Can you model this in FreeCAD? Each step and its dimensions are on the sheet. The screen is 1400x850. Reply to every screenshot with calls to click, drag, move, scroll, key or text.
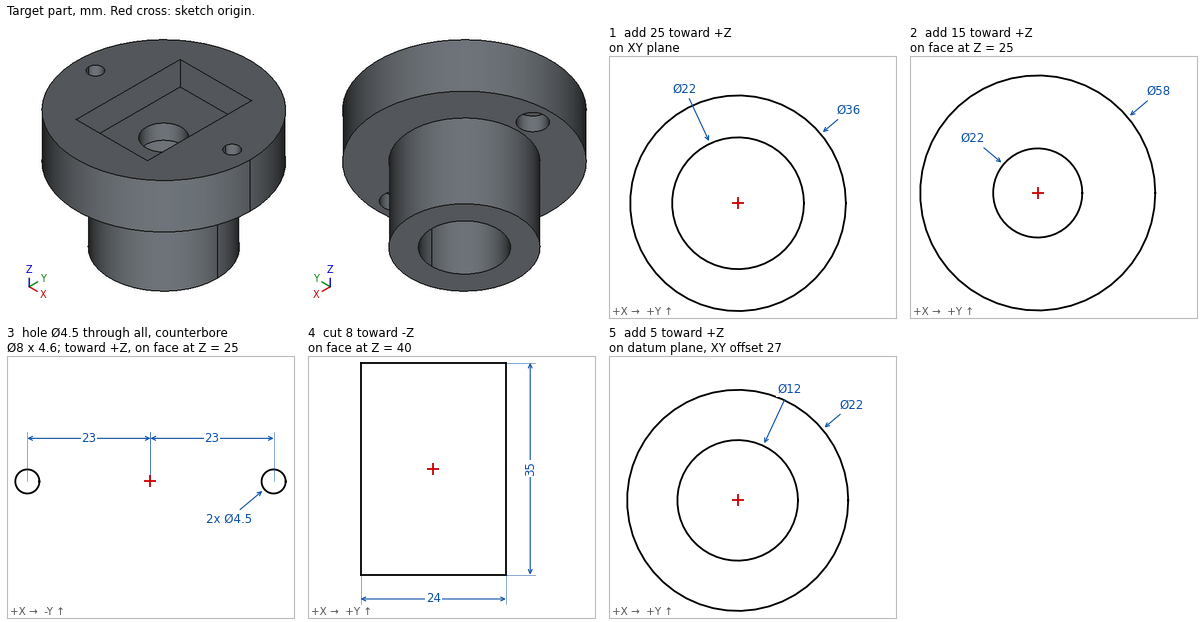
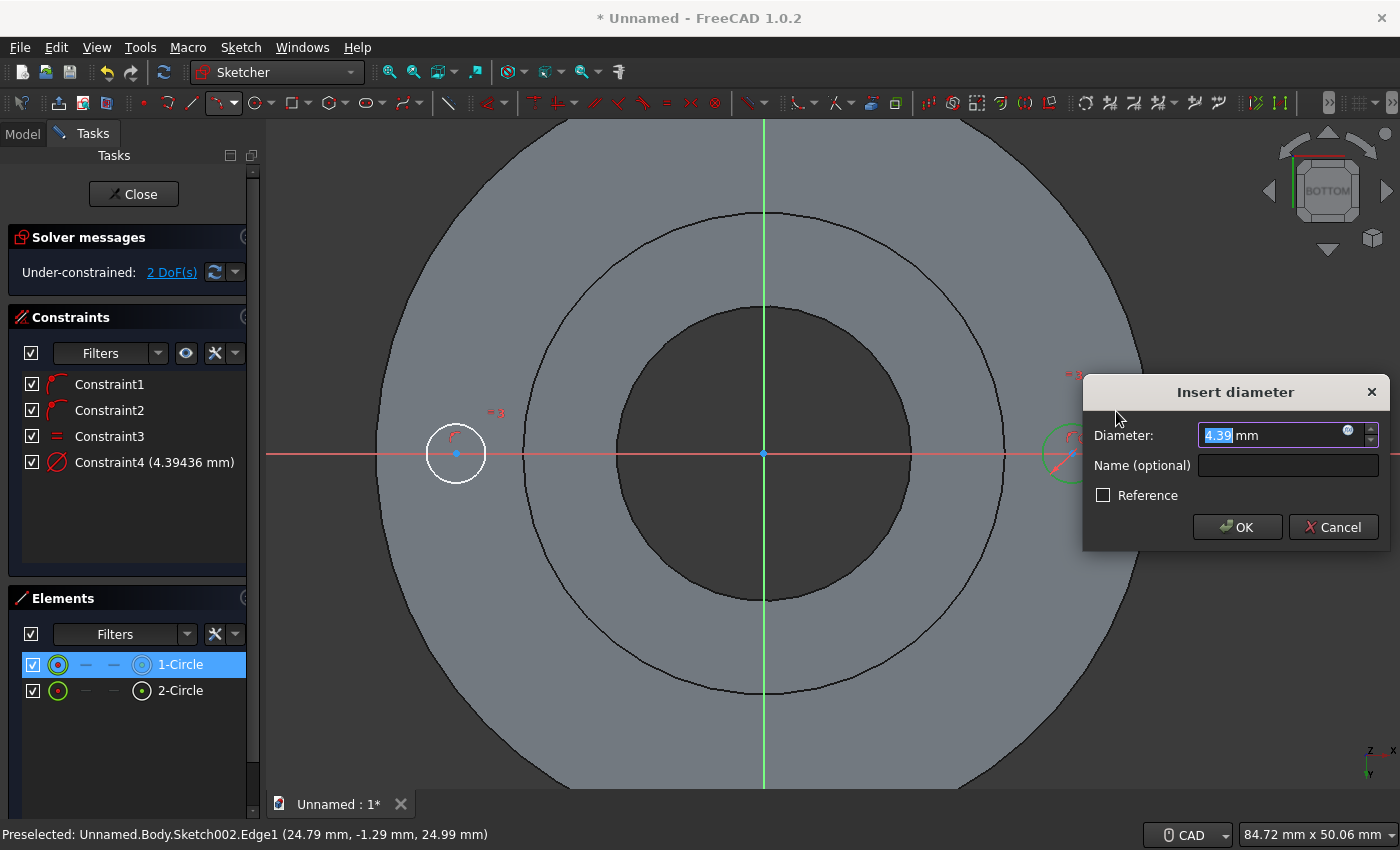
text(4.5)
key(Return)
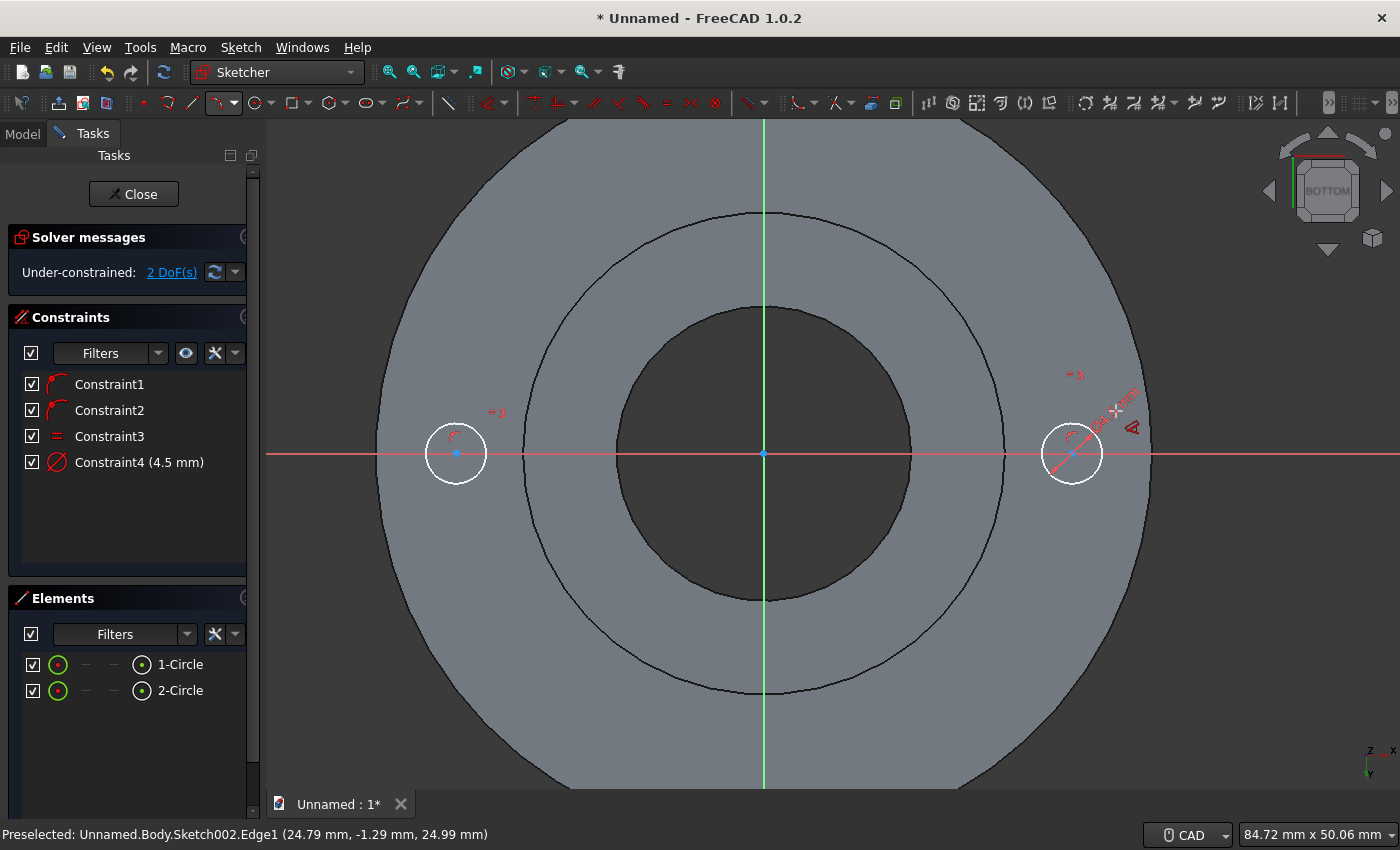
click(1072, 454)
click(918, 488)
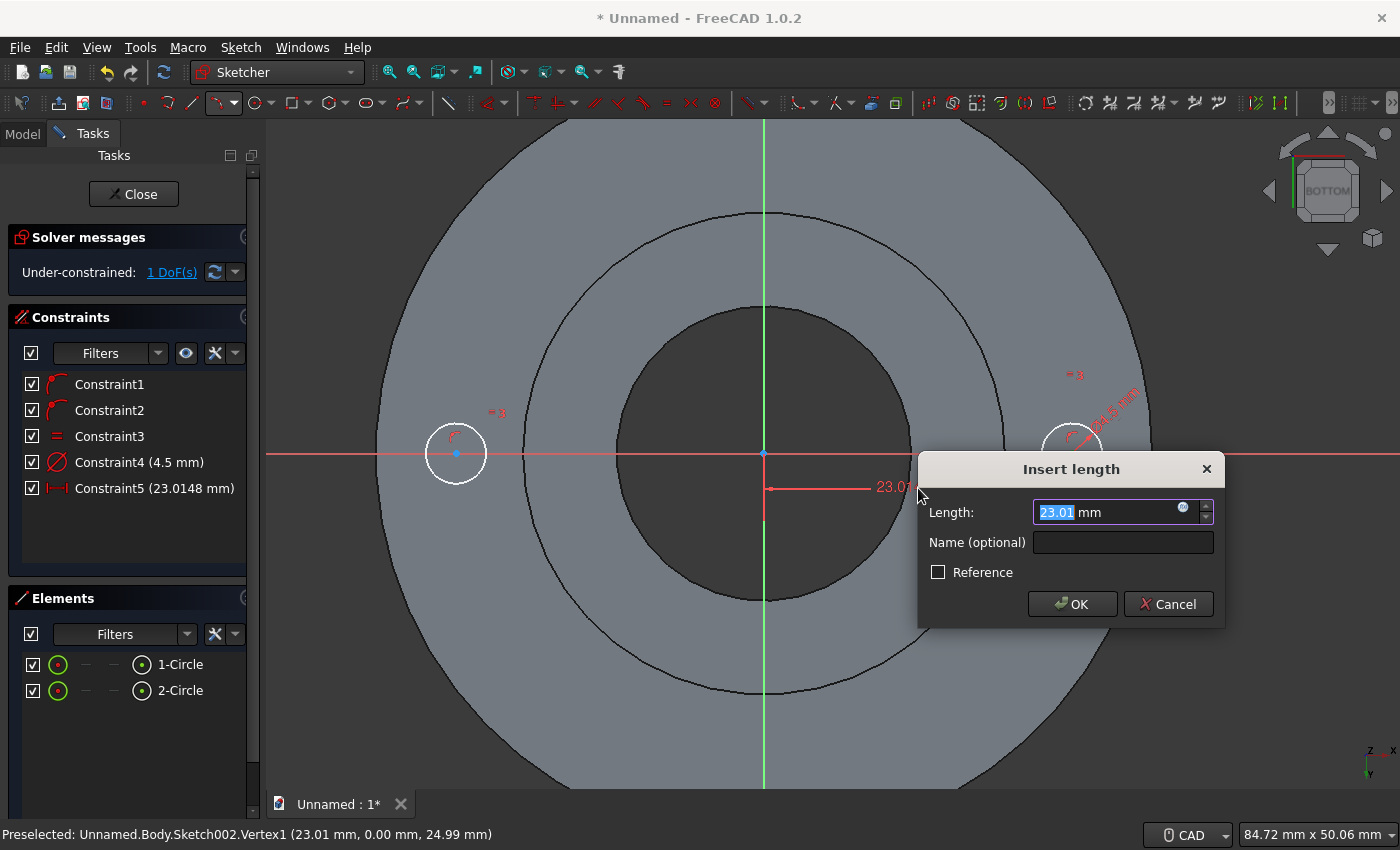
text(23)
key(Return)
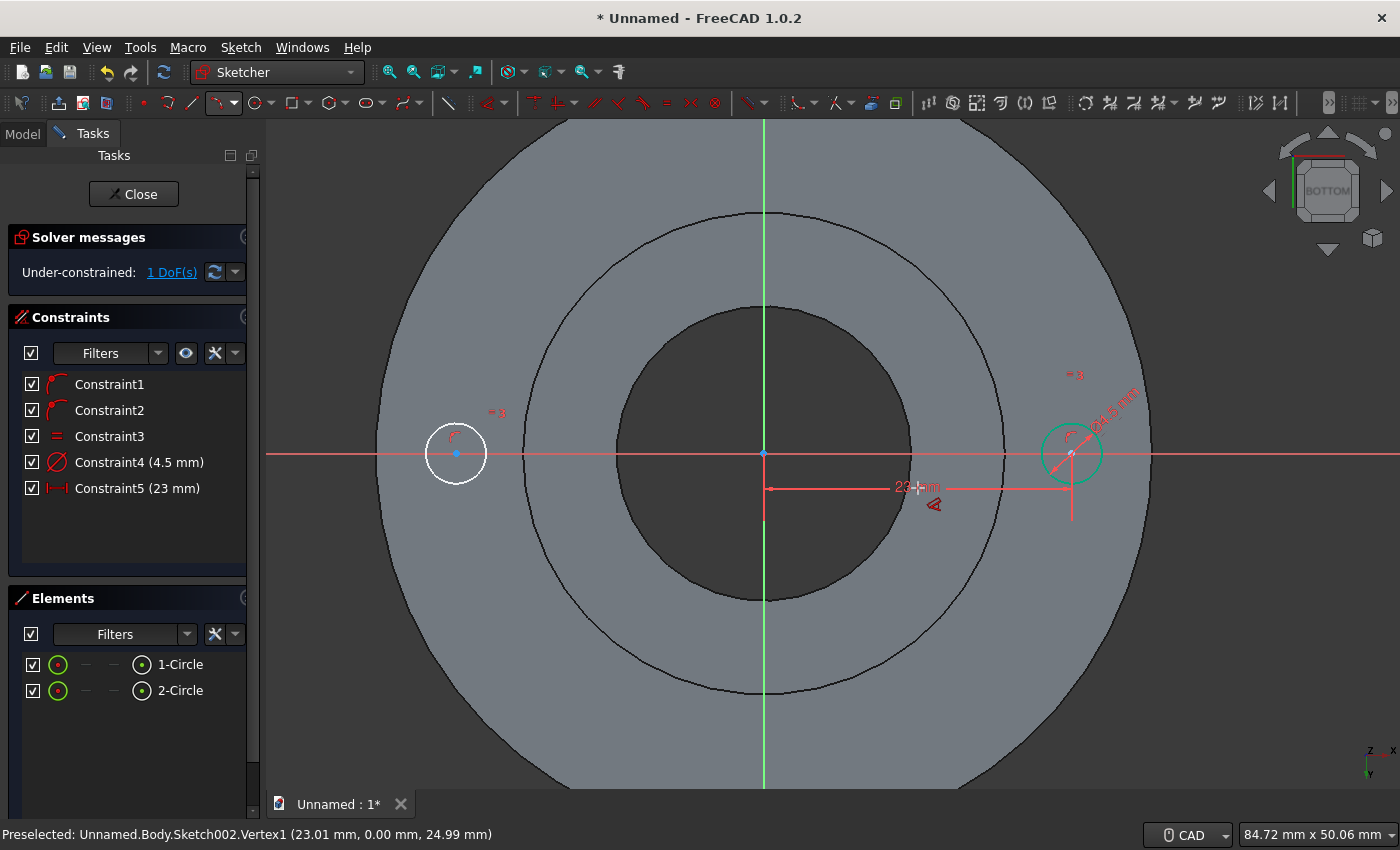
click(456, 454)
click(610, 488)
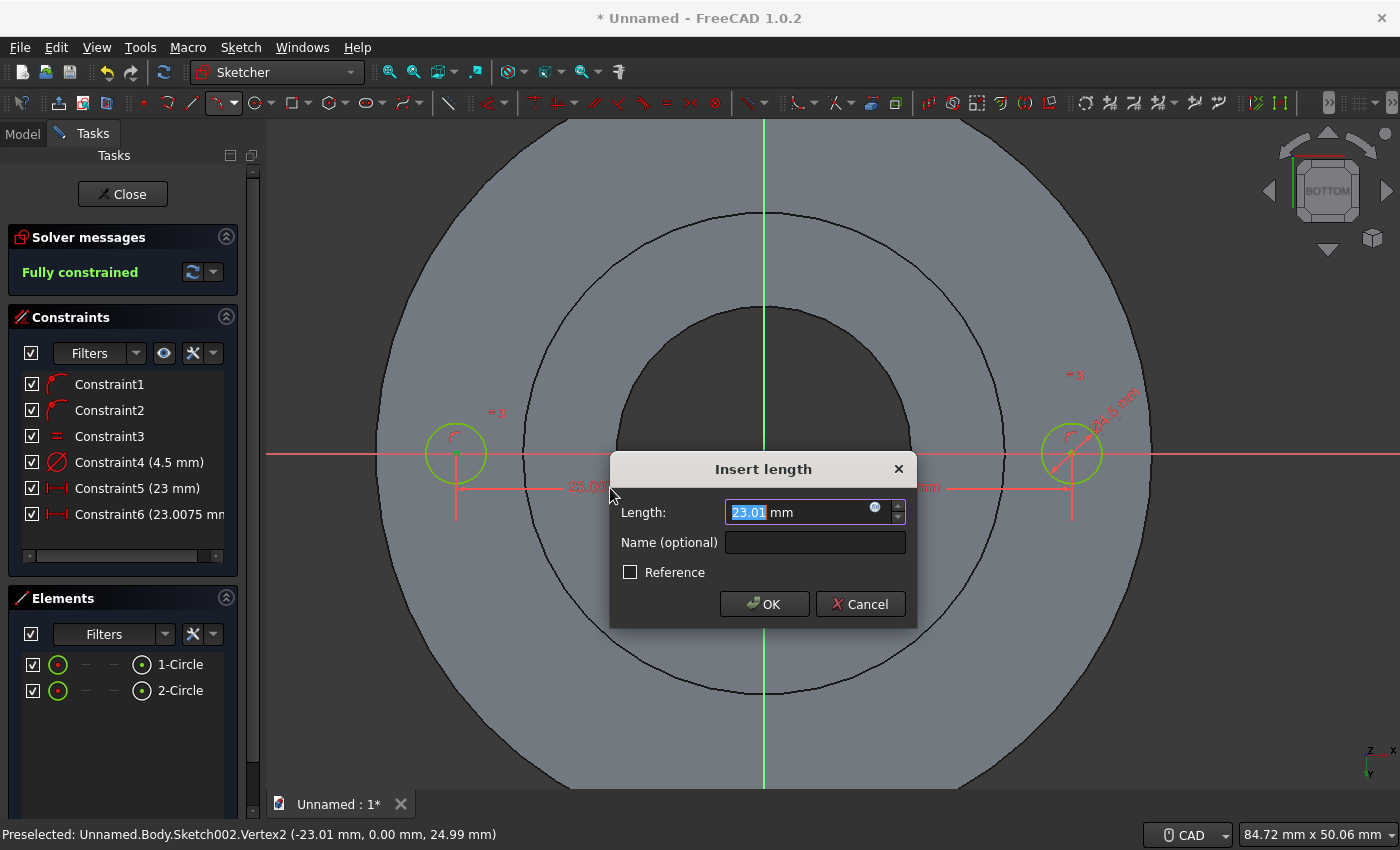
text(23)
key(Return)
key(Escape)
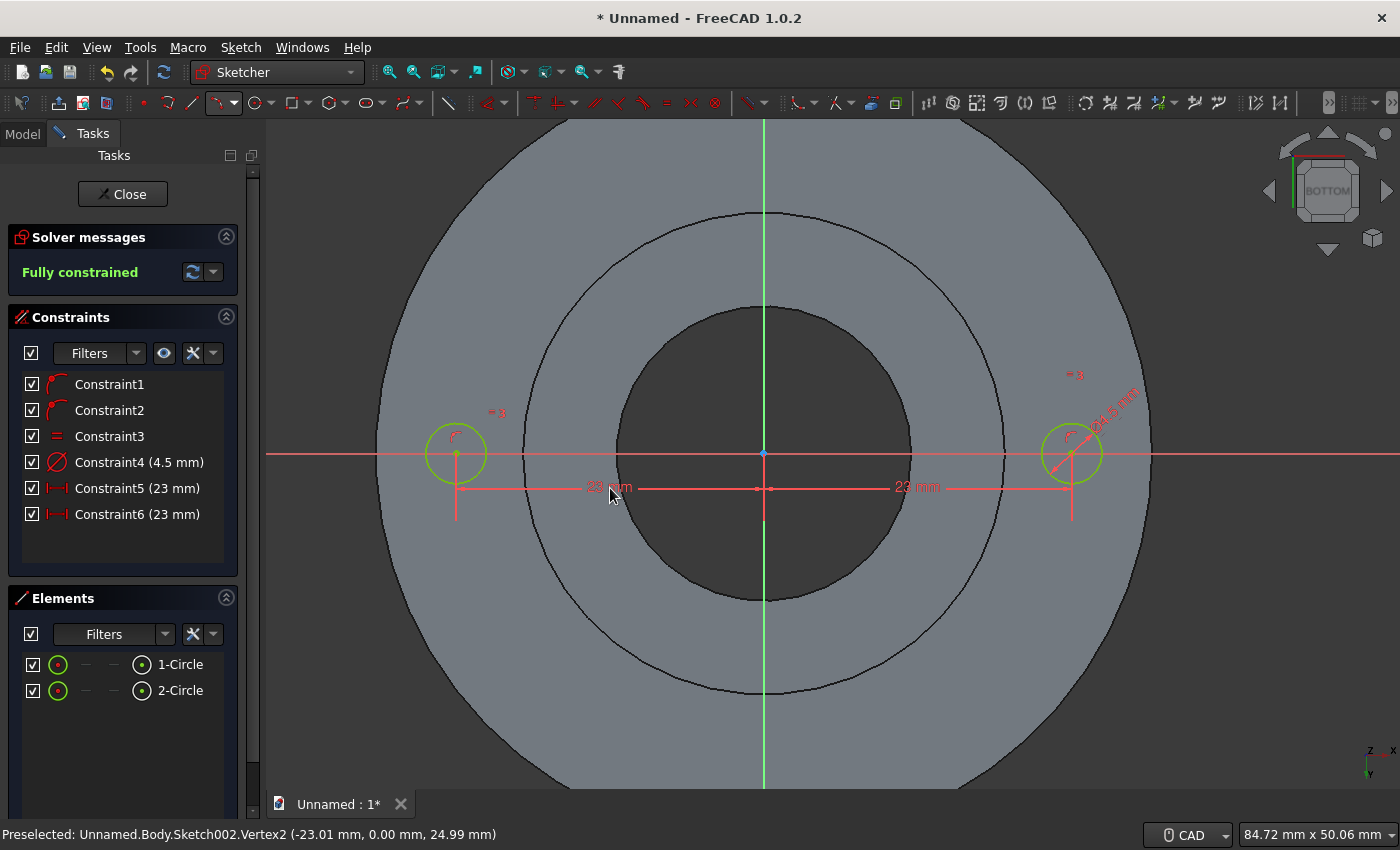
click(123, 194)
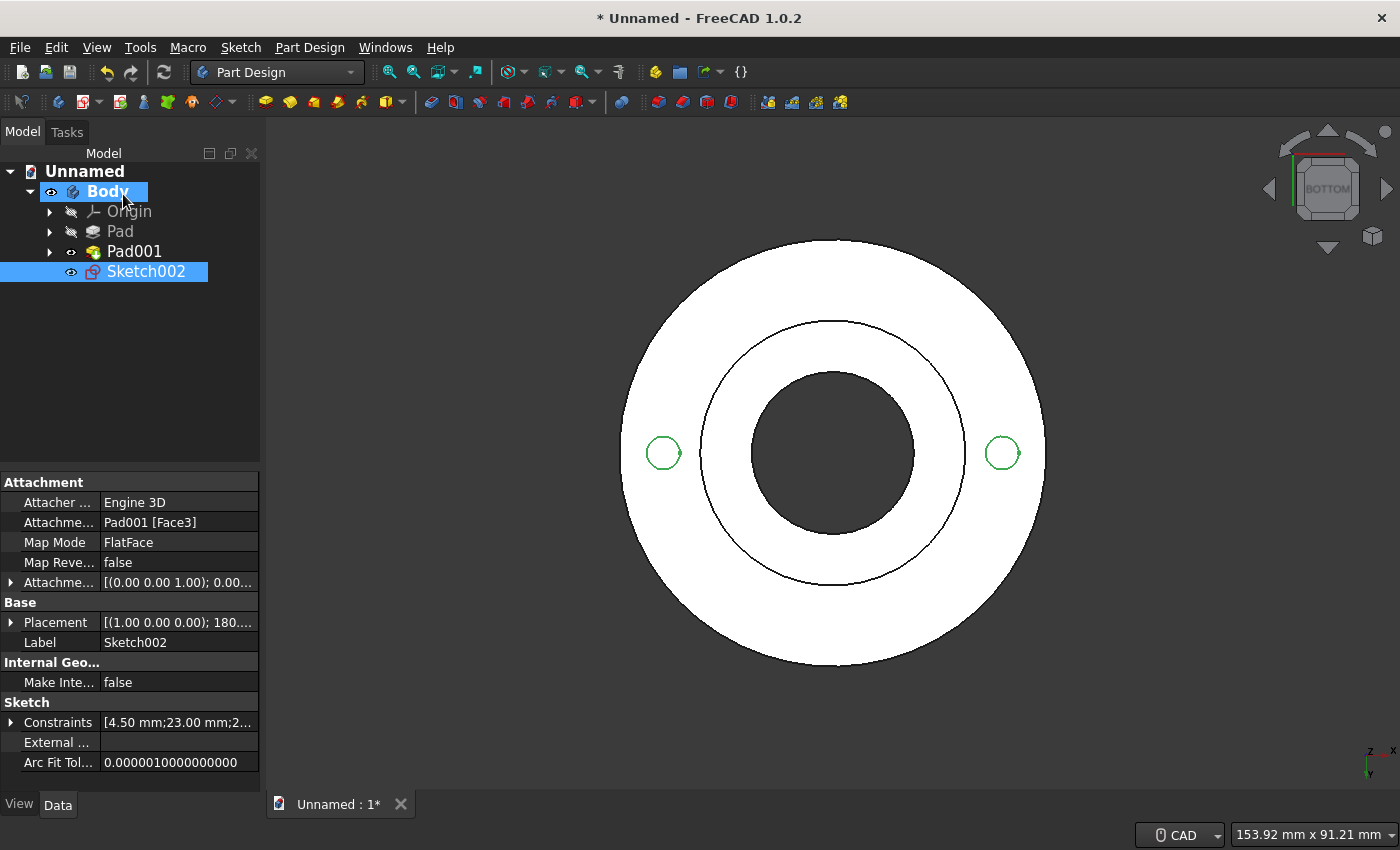
click(456, 102)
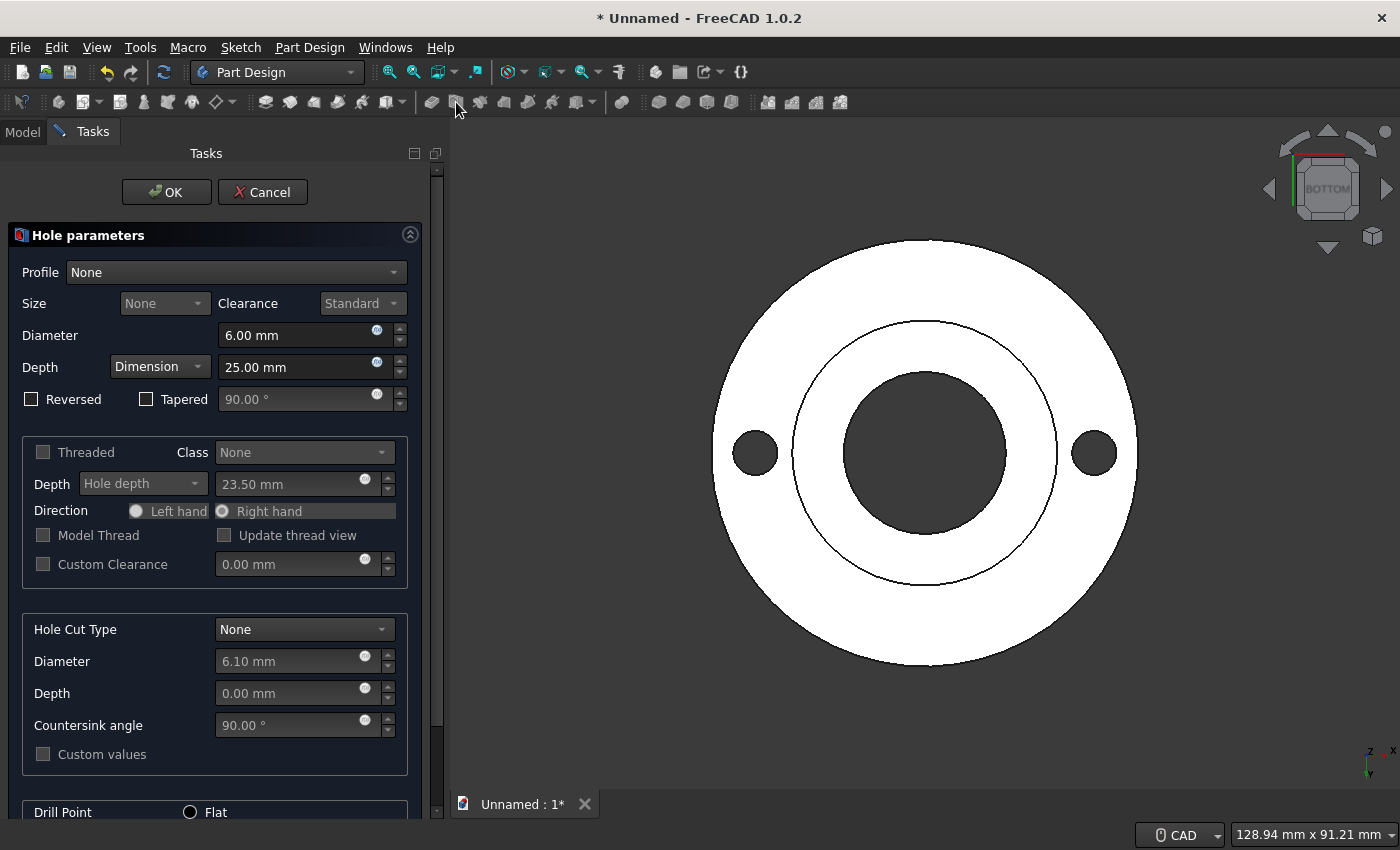
triple_click(305, 335)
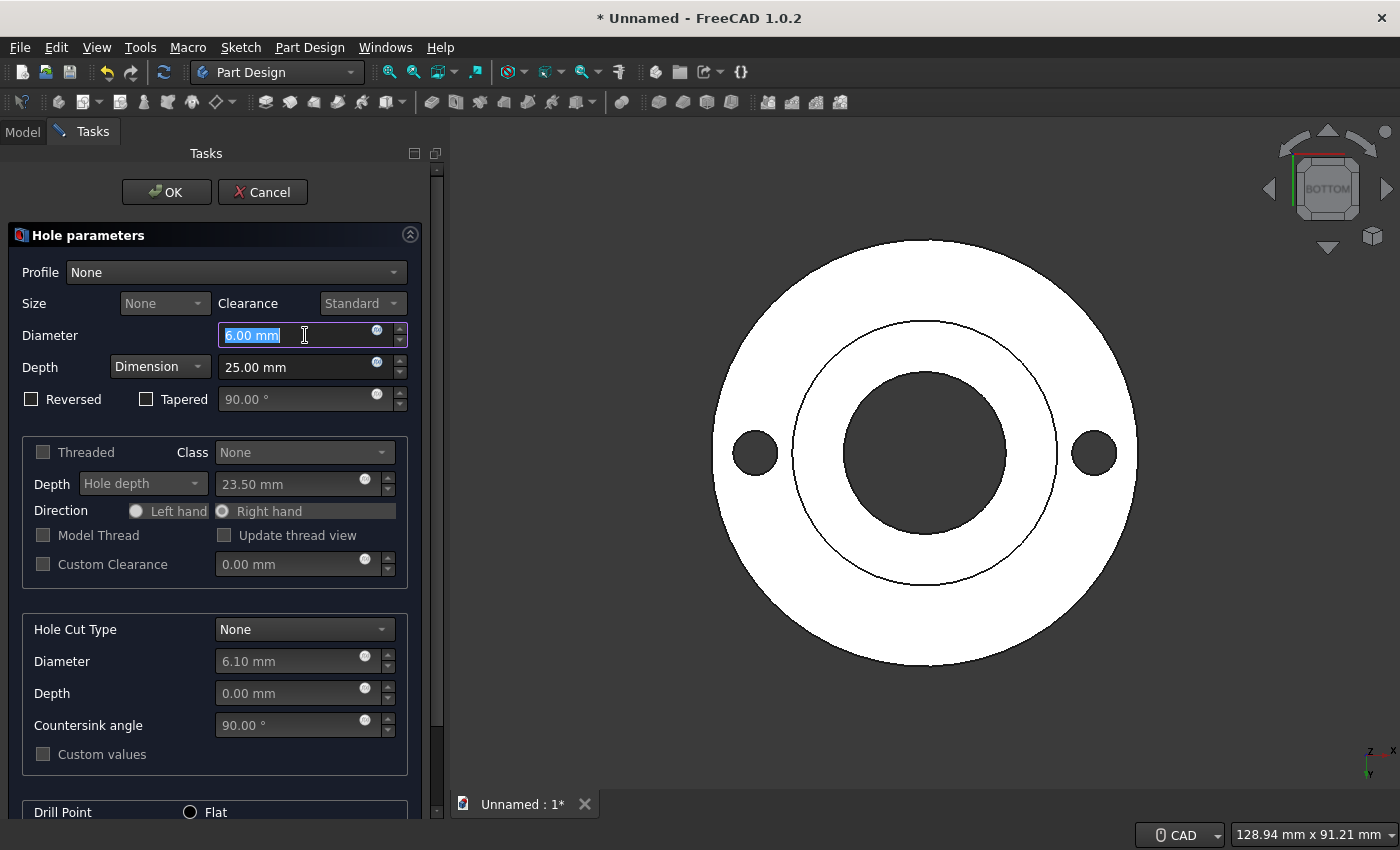
text(4.5)
key(Tab)